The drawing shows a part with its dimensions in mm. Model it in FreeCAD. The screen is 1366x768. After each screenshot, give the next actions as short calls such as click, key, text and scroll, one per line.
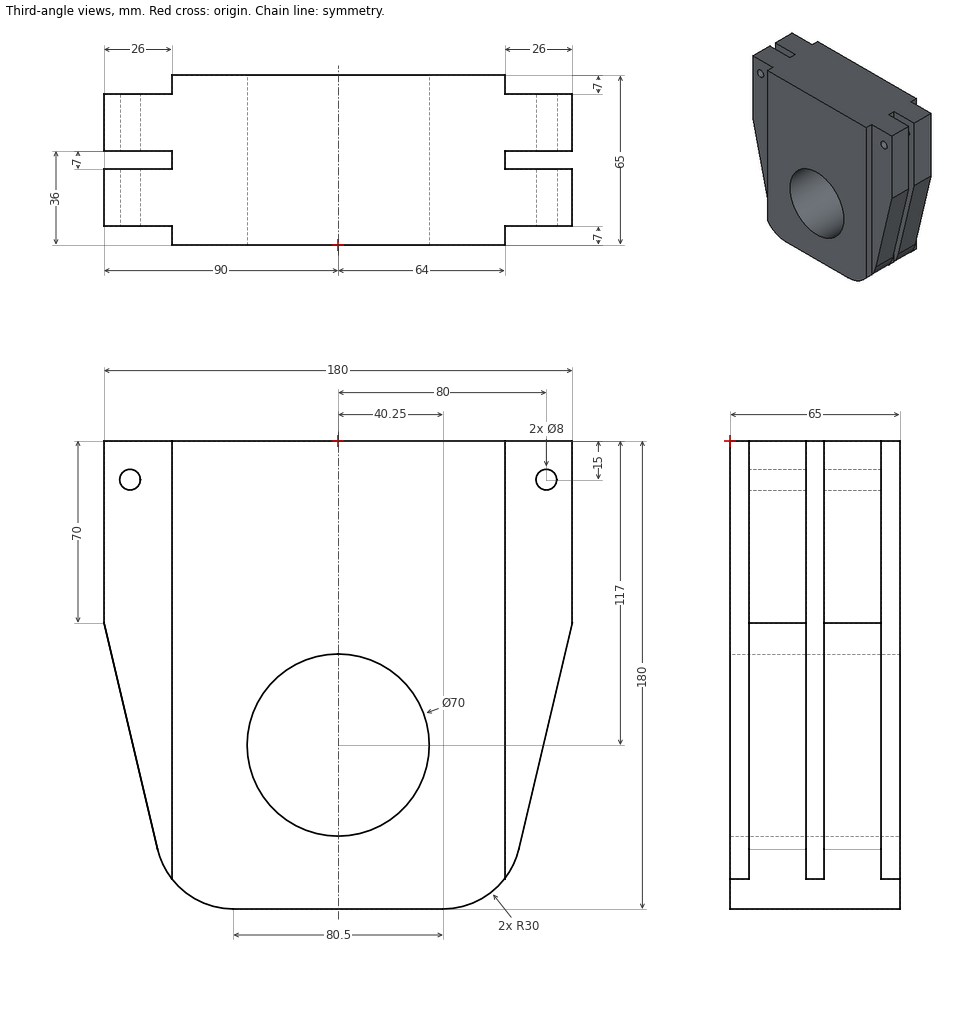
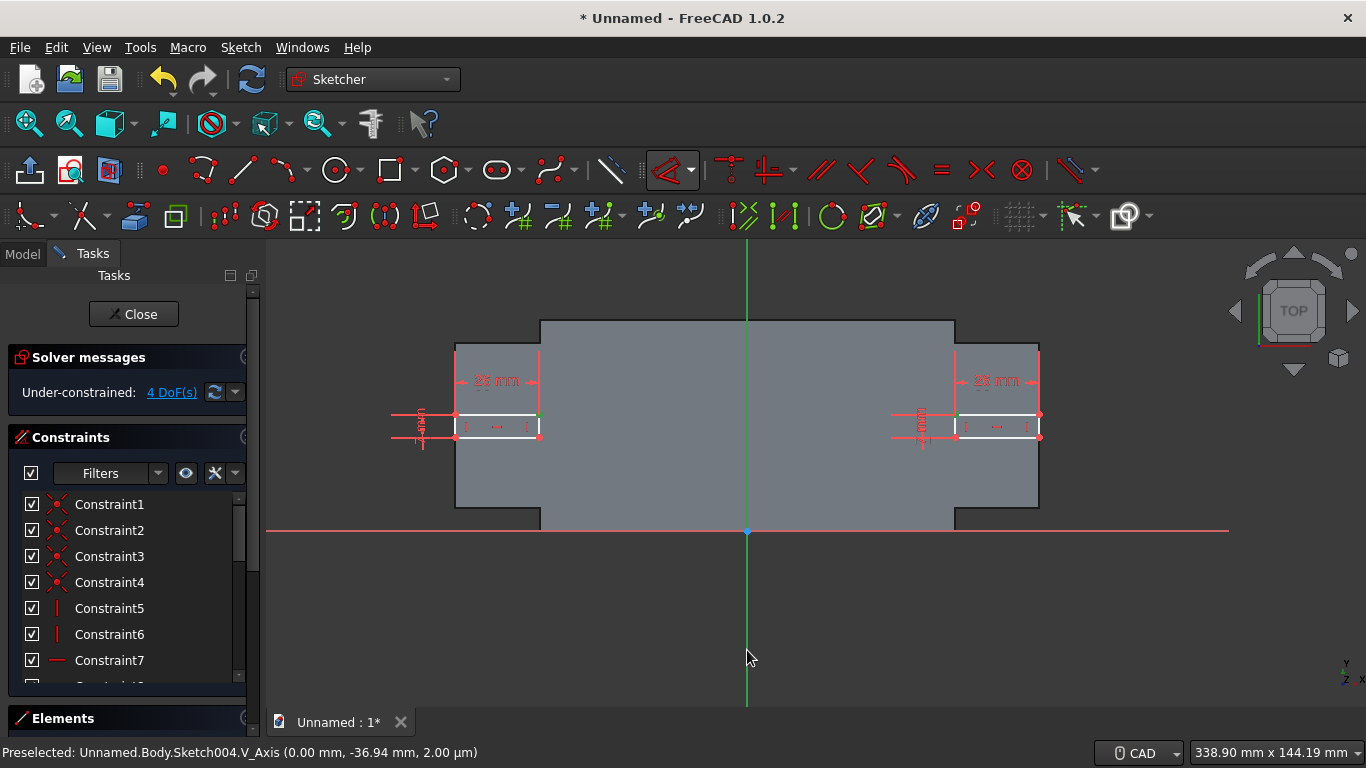
click(982, 170)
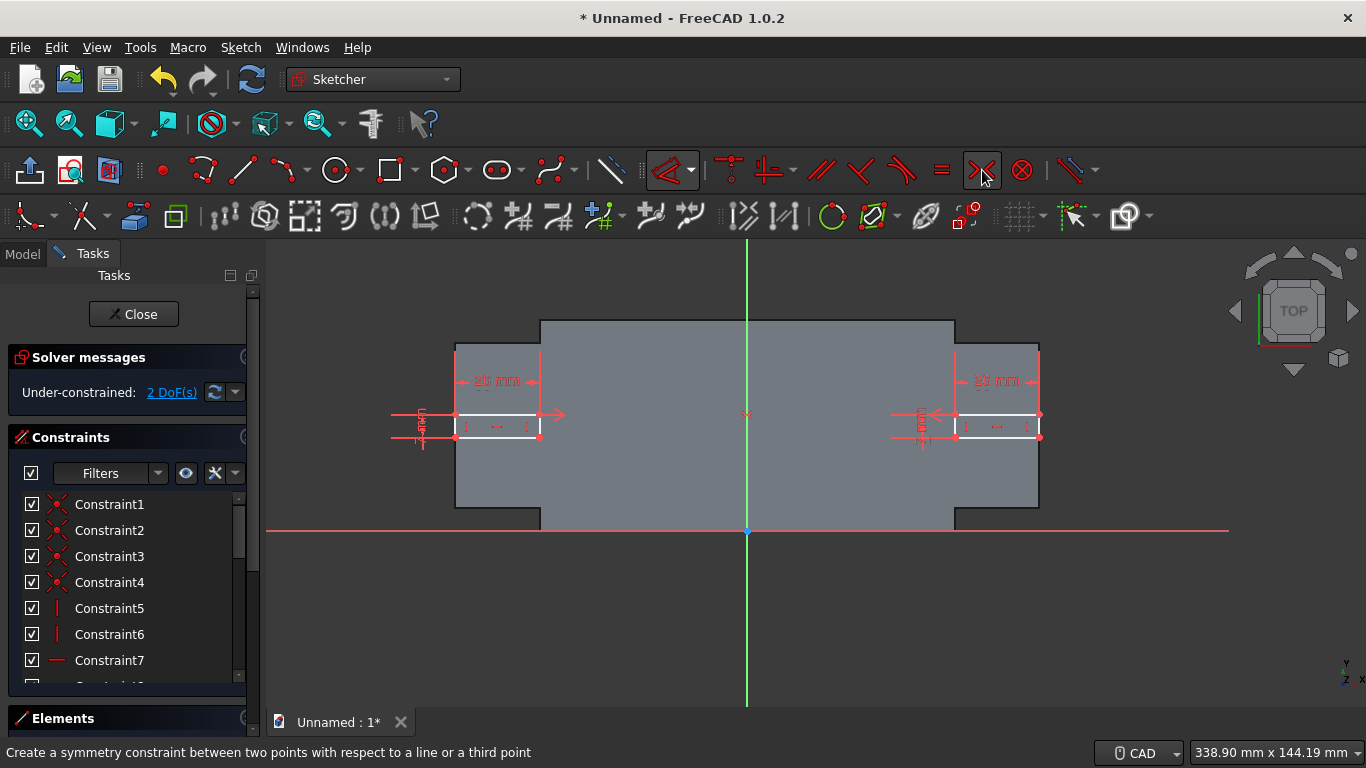
click(455, 415)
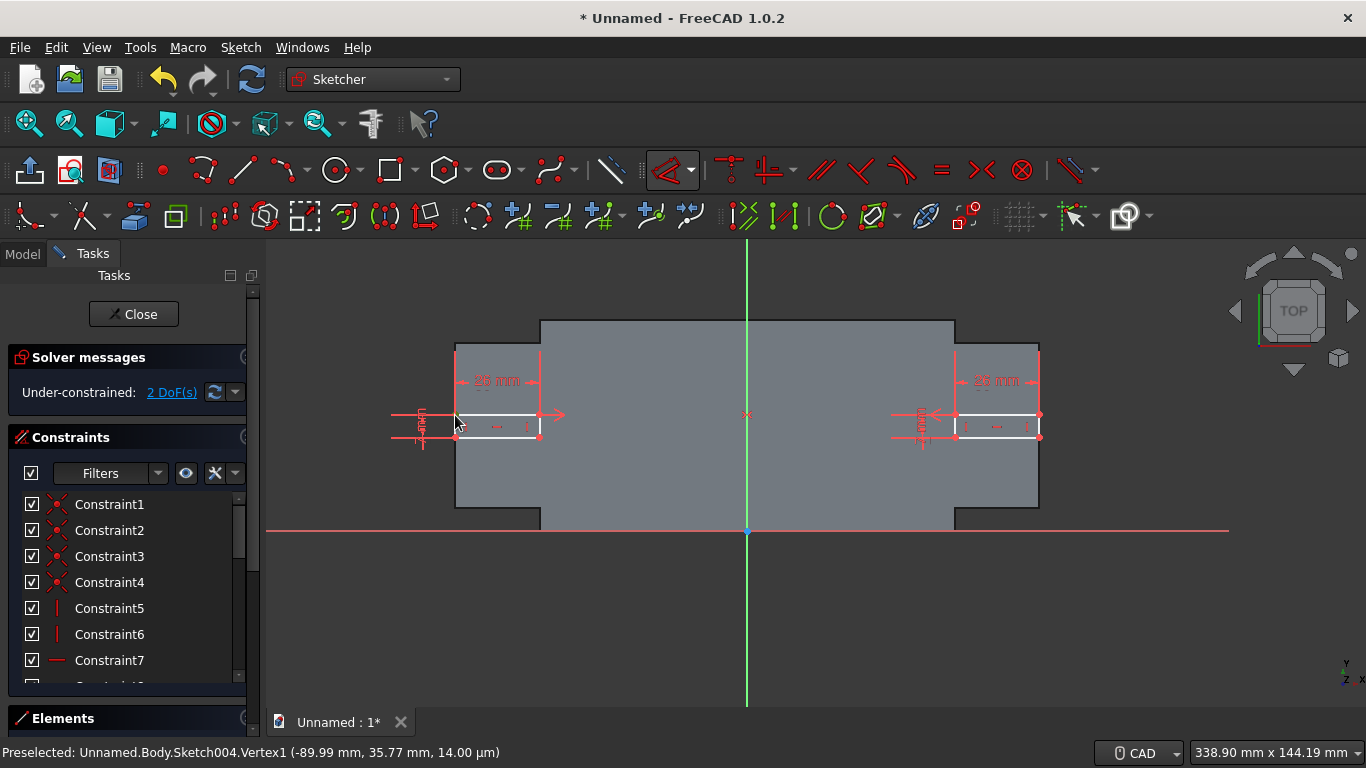
click(694, 170)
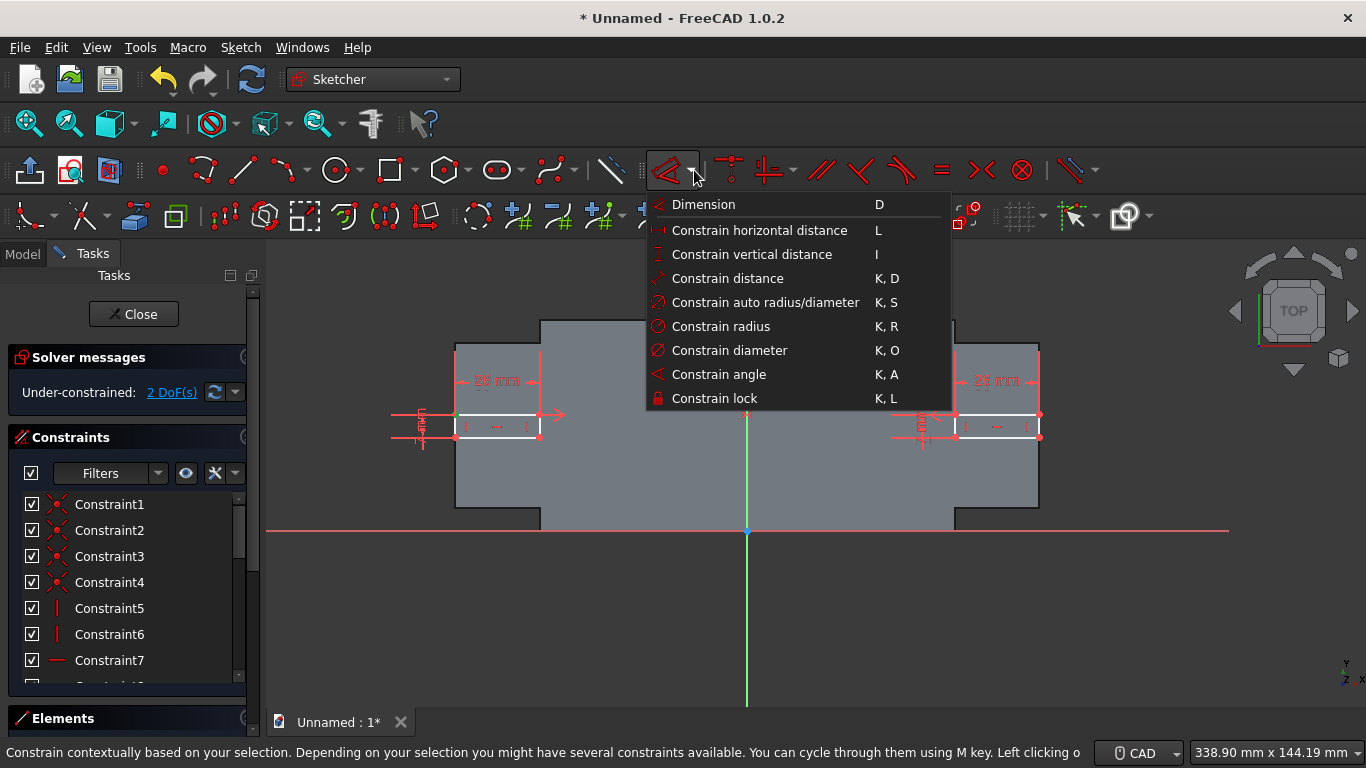
click(799, 230)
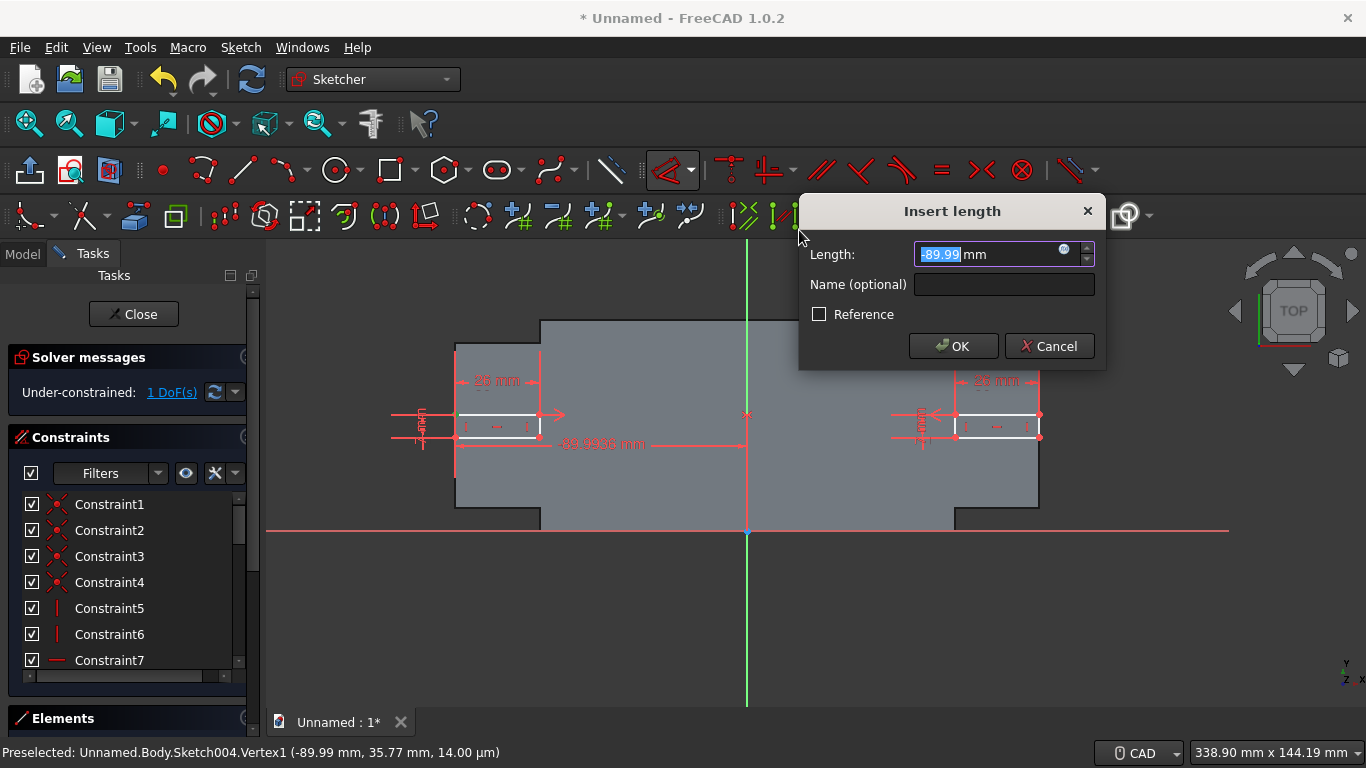
text(-90)
key(Return)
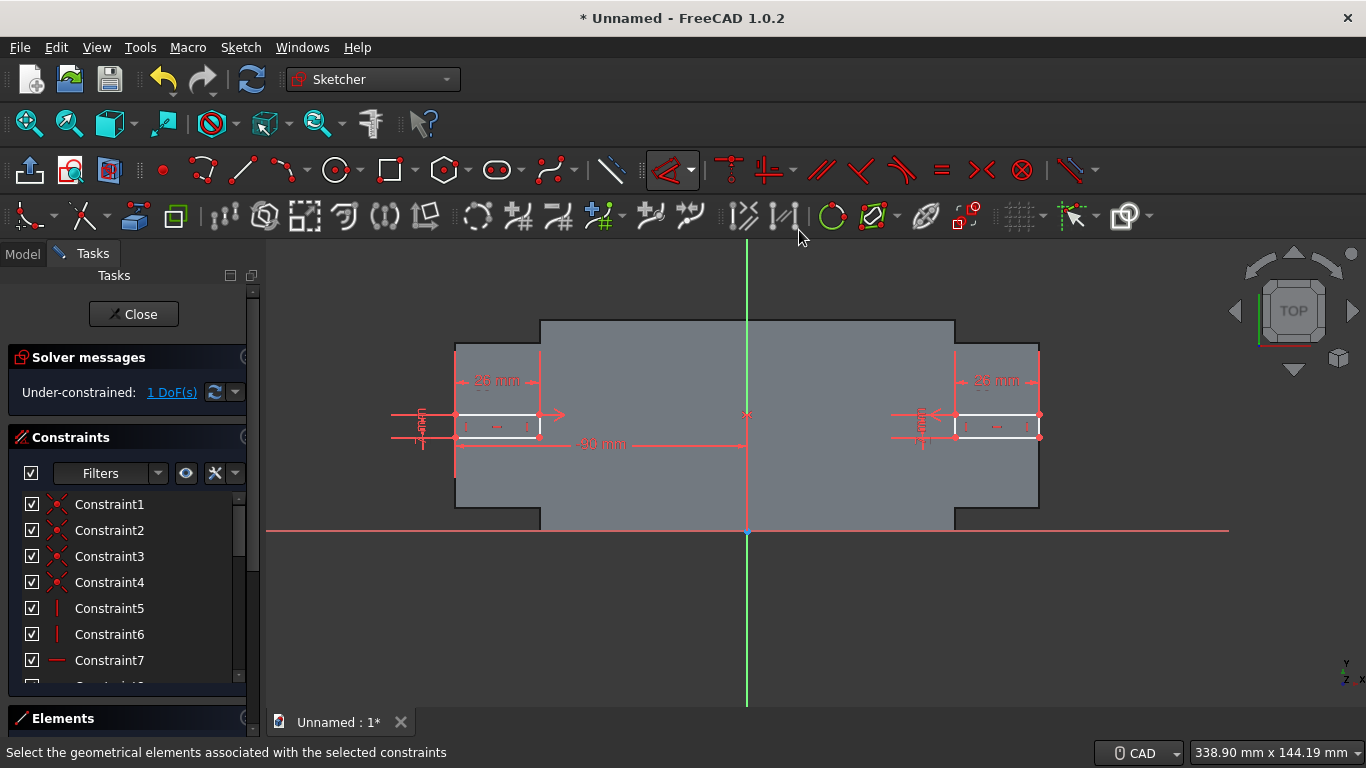
click(455, 415)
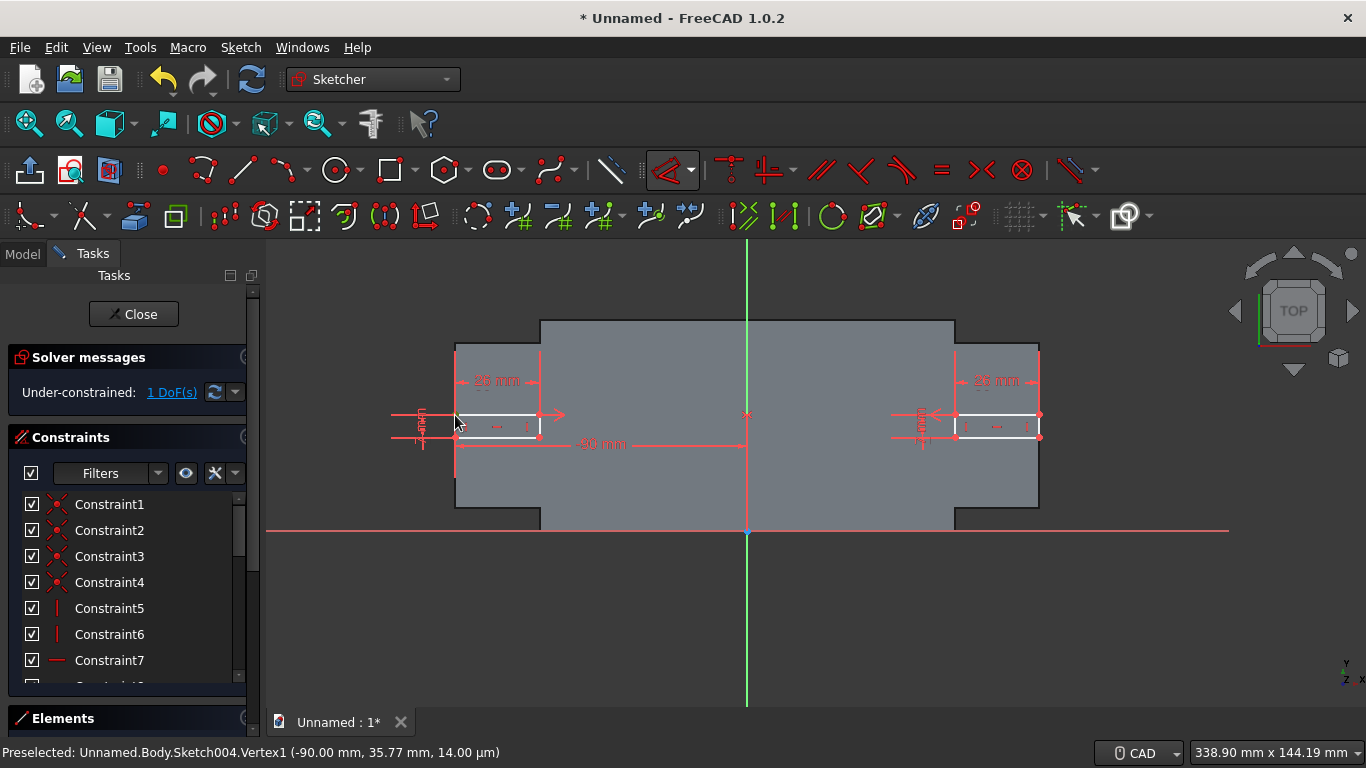
key(i)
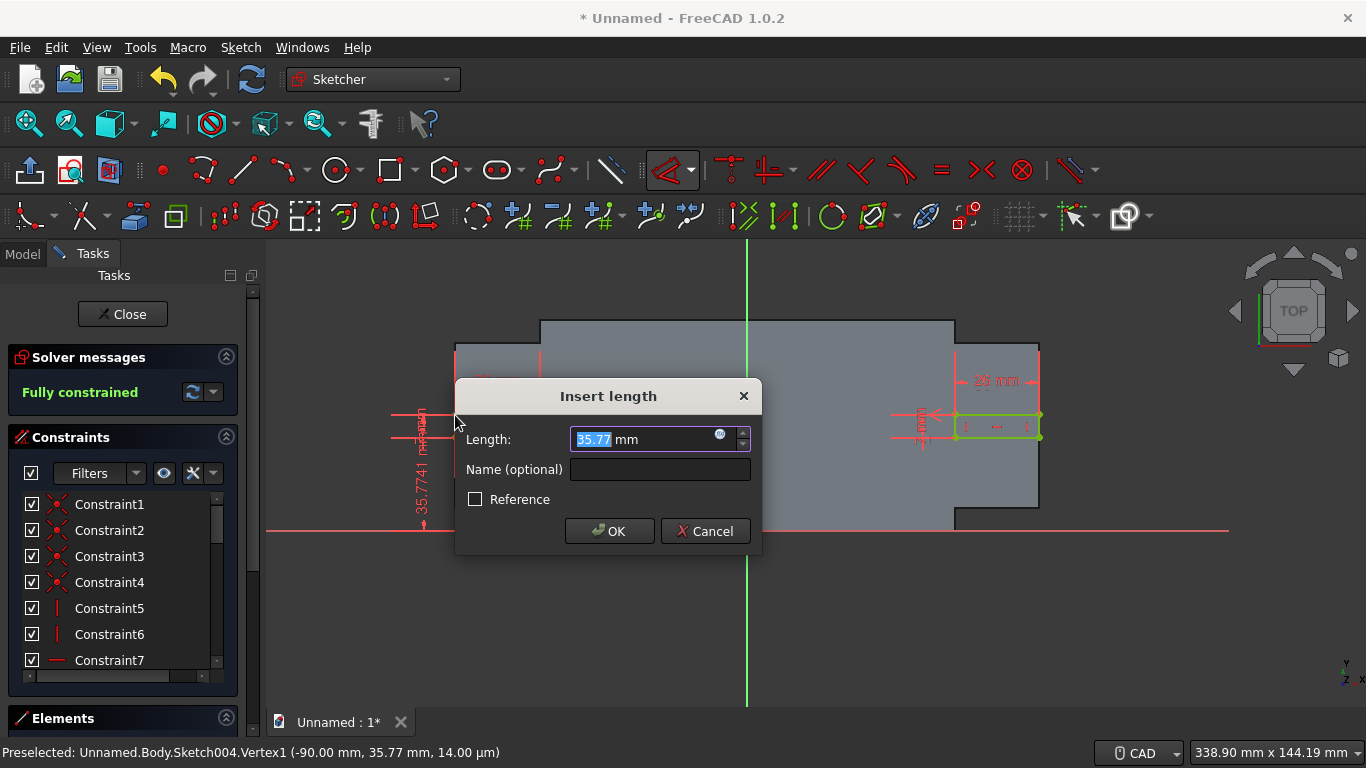
text(36)
key(Return)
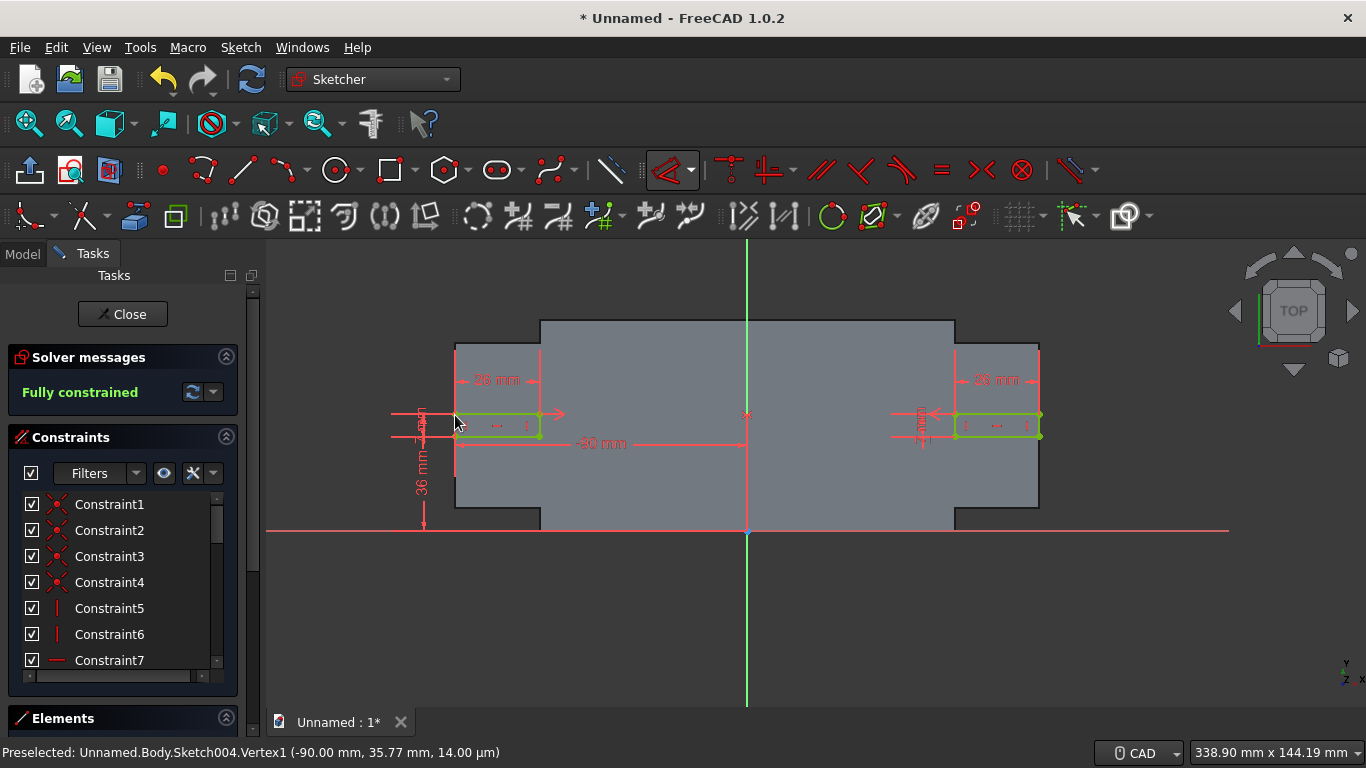
click(123, 314)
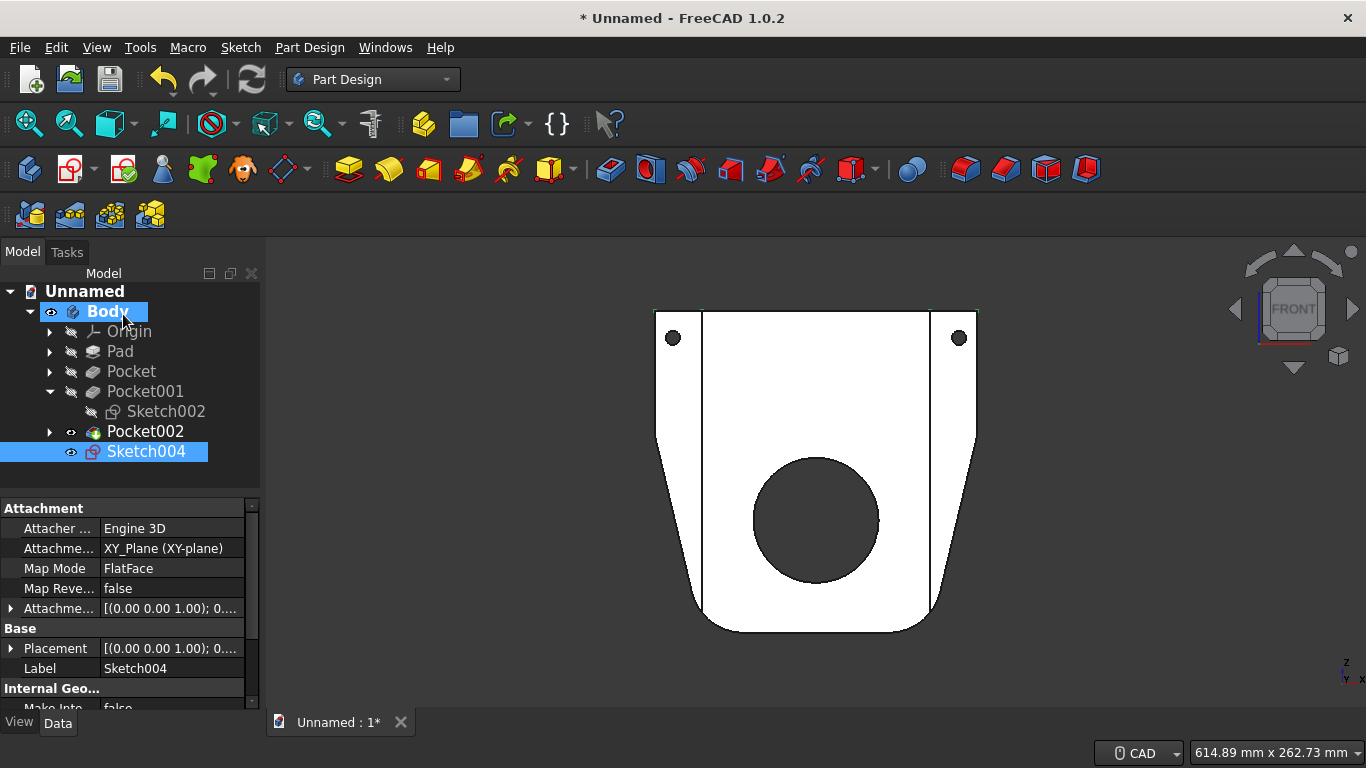
click(612, 170)